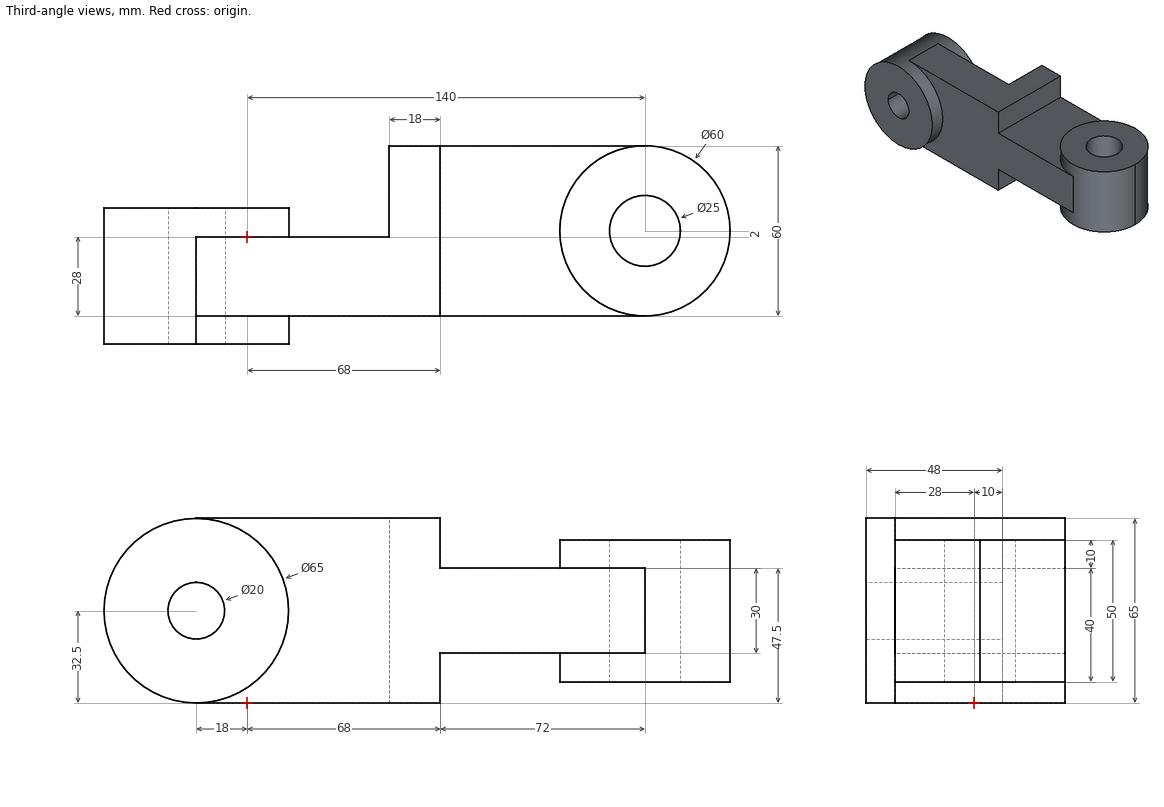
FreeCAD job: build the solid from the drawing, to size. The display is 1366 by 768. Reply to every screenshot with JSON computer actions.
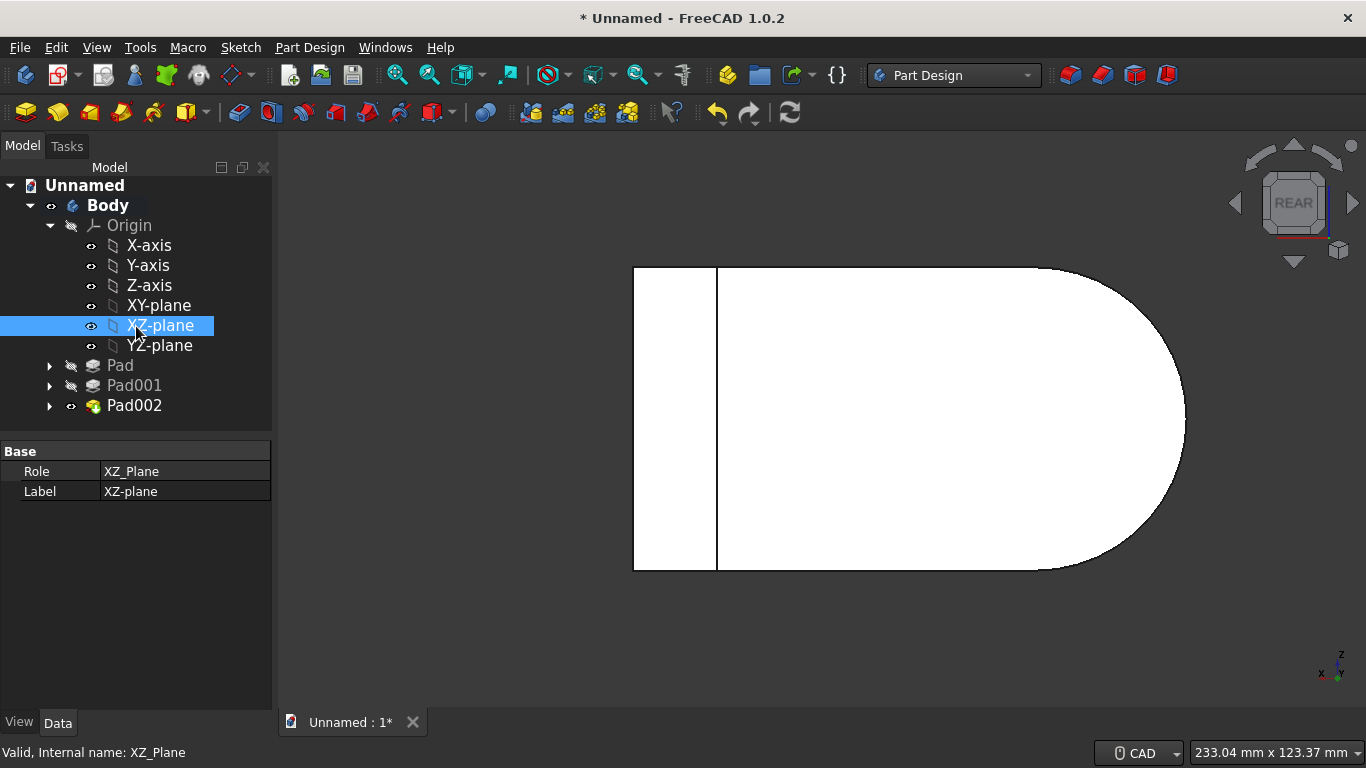
{"action": "left_click", "coordinate": [232, 76]}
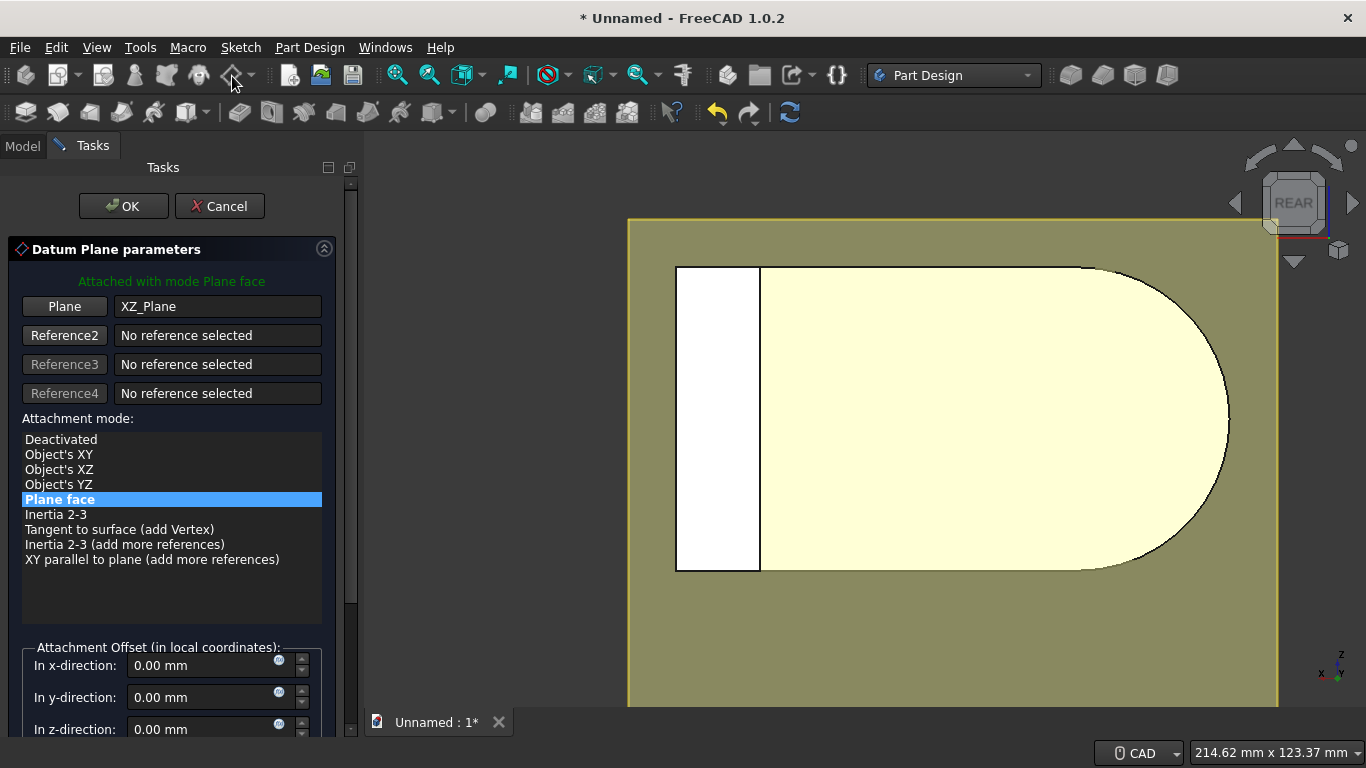
{"action": "scroll", "coordinate": [351, 456], "scroll_direction": "down", "scroll_amount": 2}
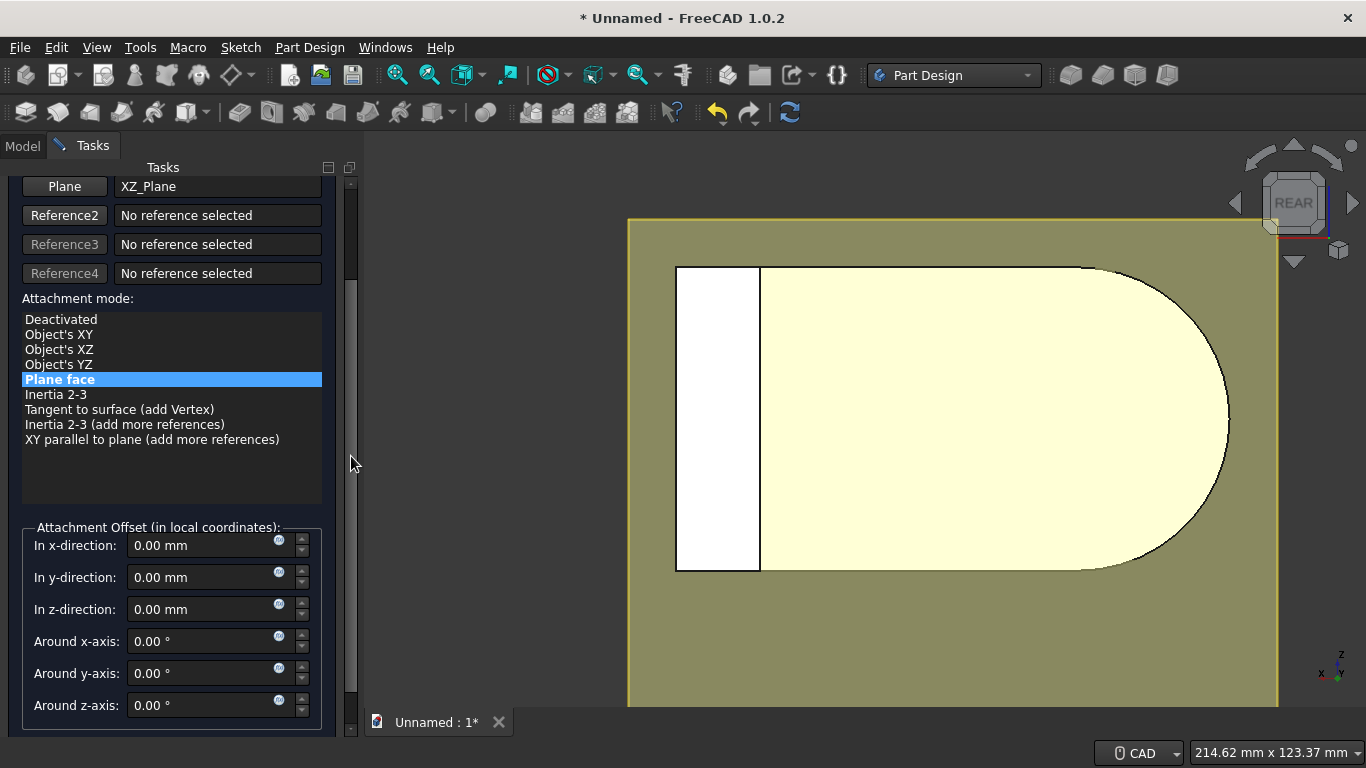
{"action": "triple_click", "coordinate": [210, 609]}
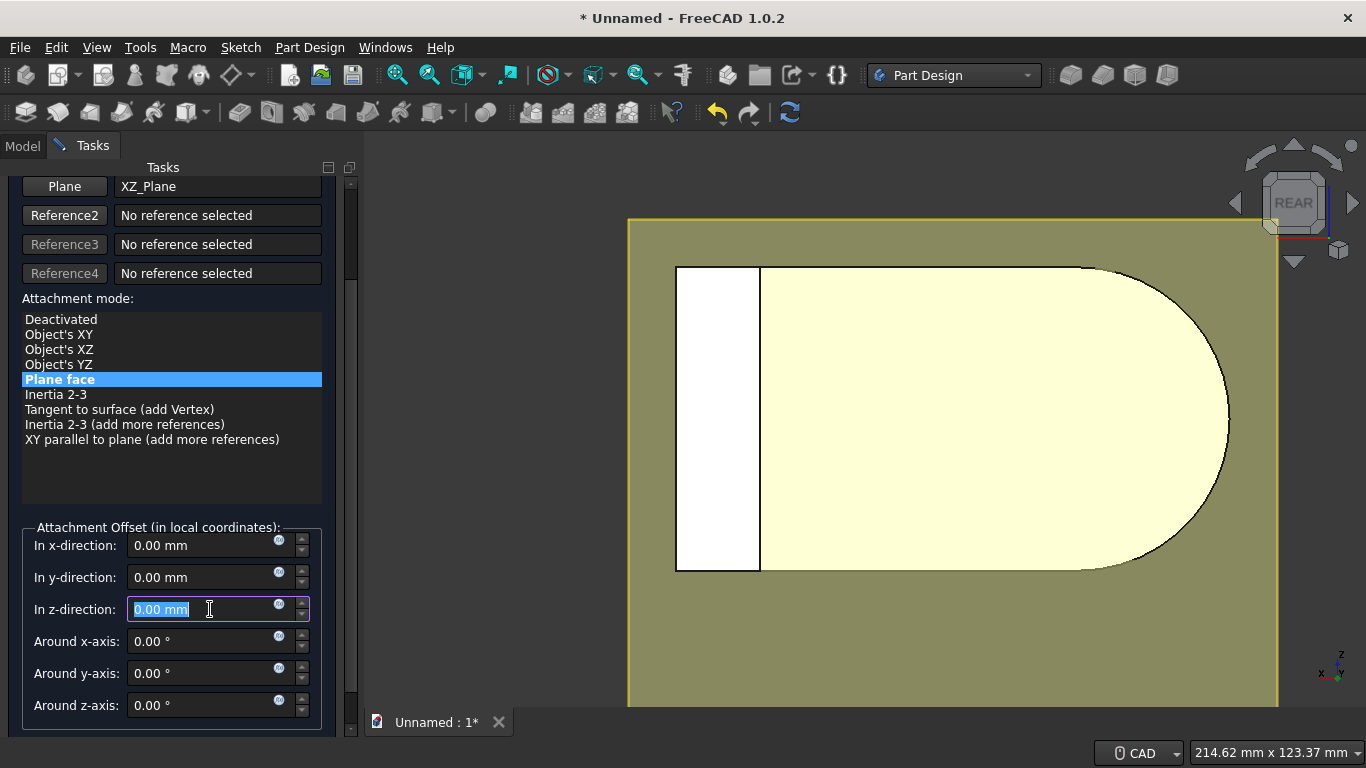
{"action": "type", "text": "-10"}
{"action": "key", "text": "Tab"}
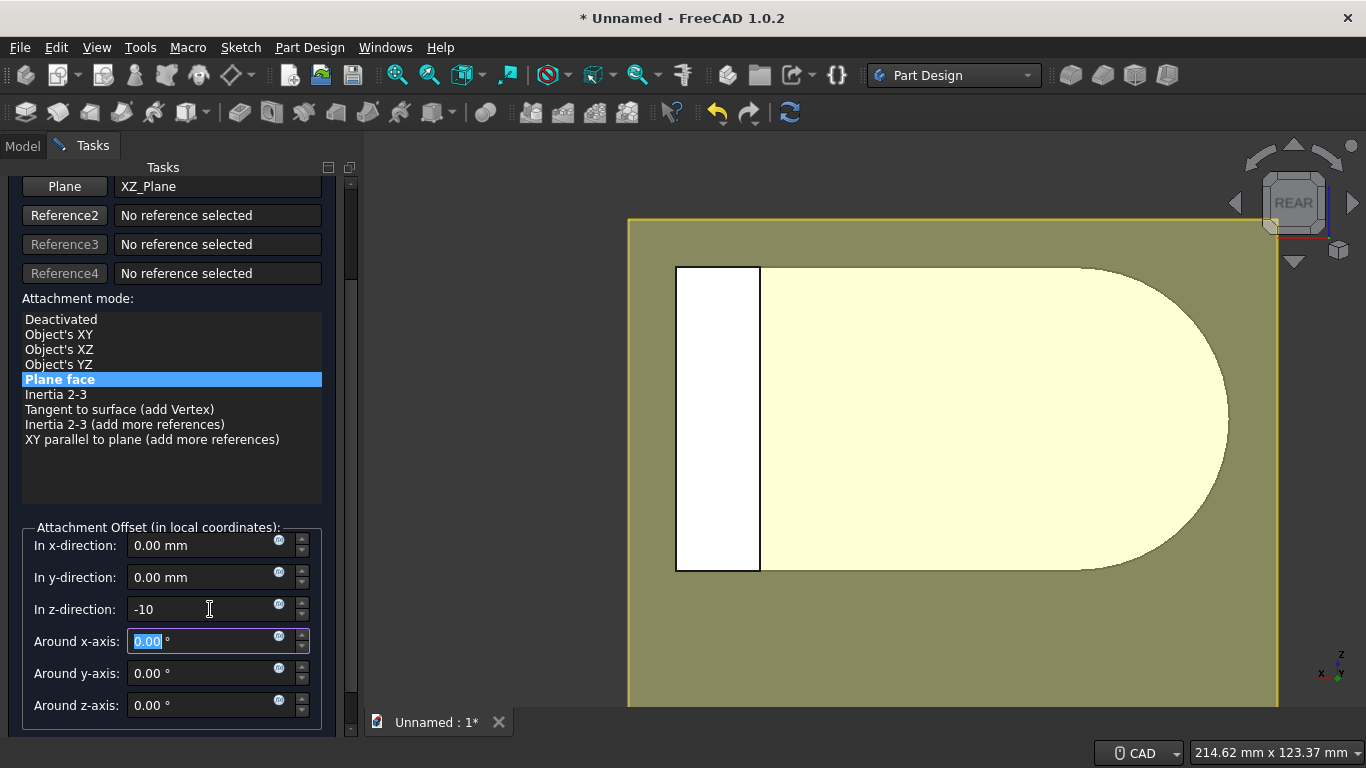
{"action": "scroll", "coordinate": [351, 456], "scroll_direction": "up", "scroll_amount": 3}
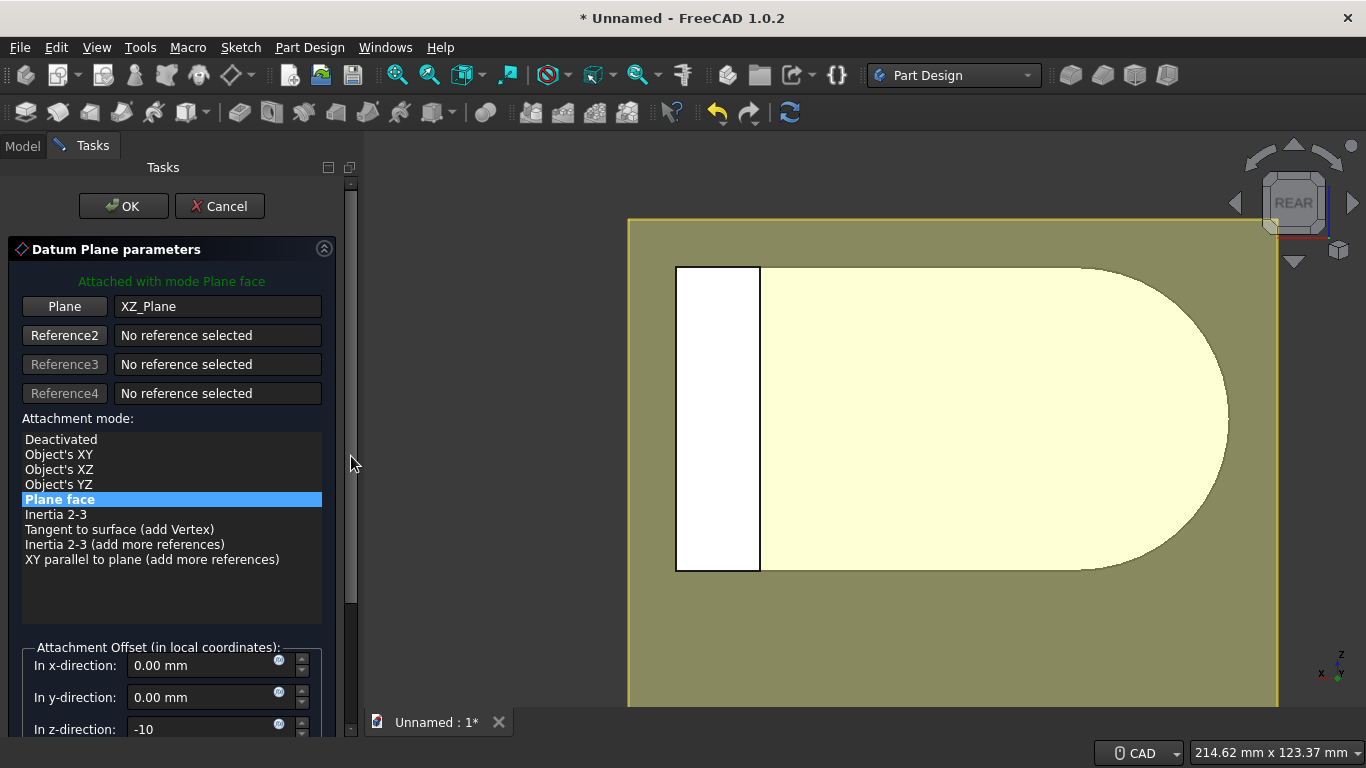
{"action": "left_click", "coordinate": [124, 206]}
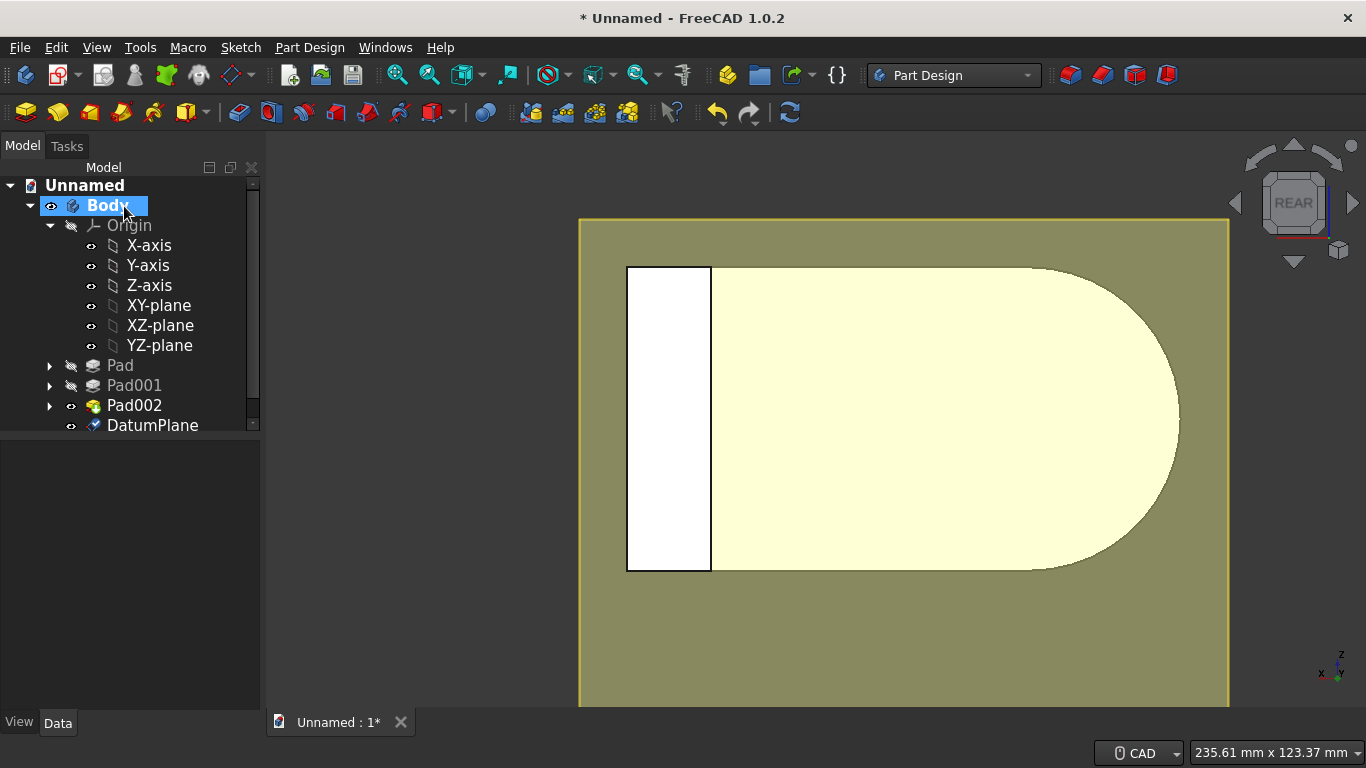
{"action": "left_click", "coordinate": [116, 426]}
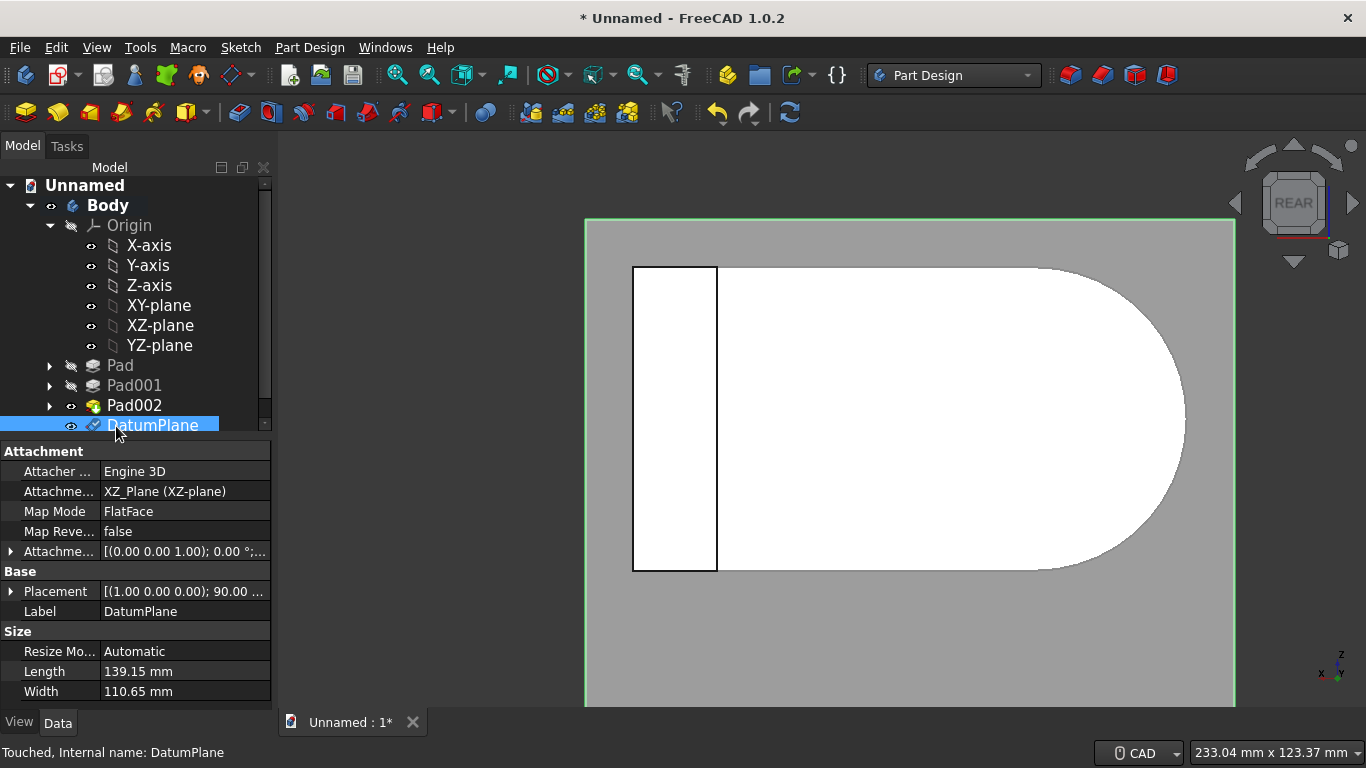
{"action": "left_click", "coordinate": [58, 76]}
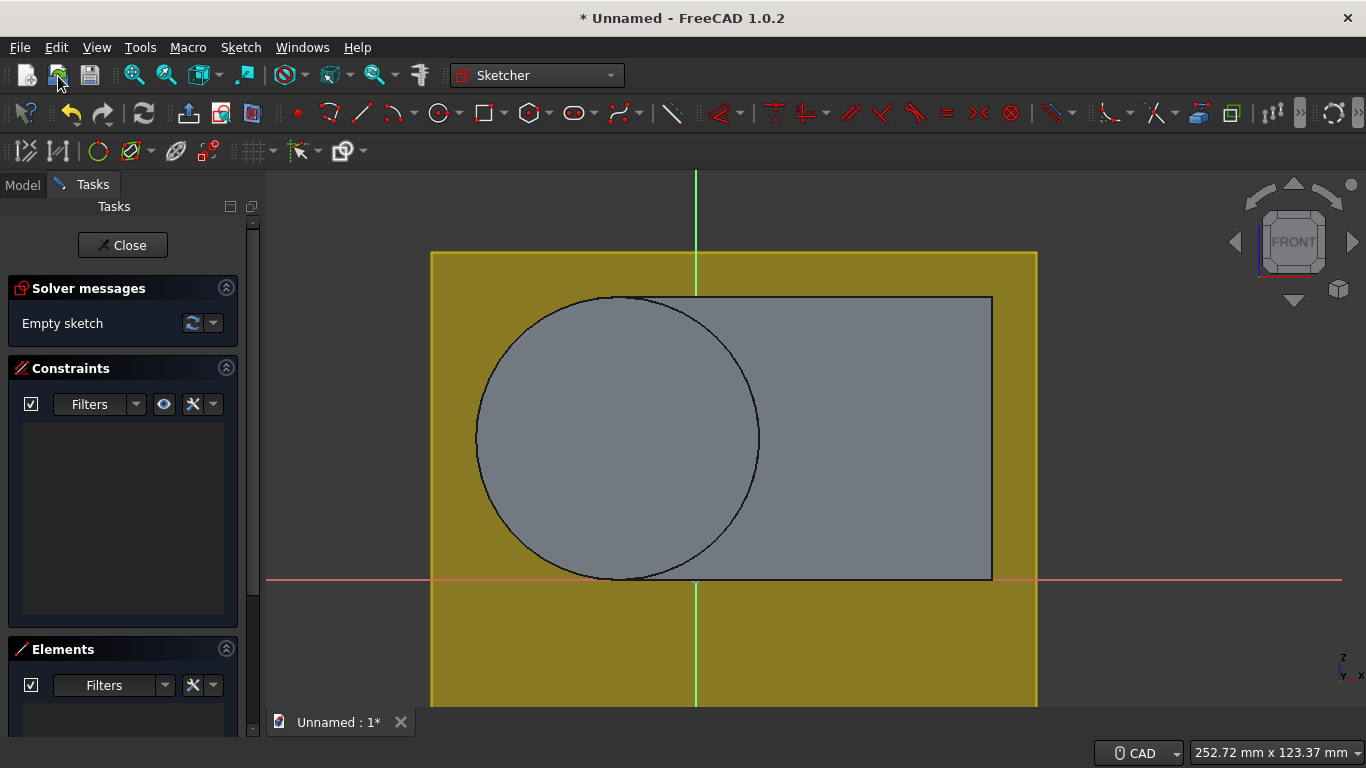
{"action": "key", "text": "q s"}